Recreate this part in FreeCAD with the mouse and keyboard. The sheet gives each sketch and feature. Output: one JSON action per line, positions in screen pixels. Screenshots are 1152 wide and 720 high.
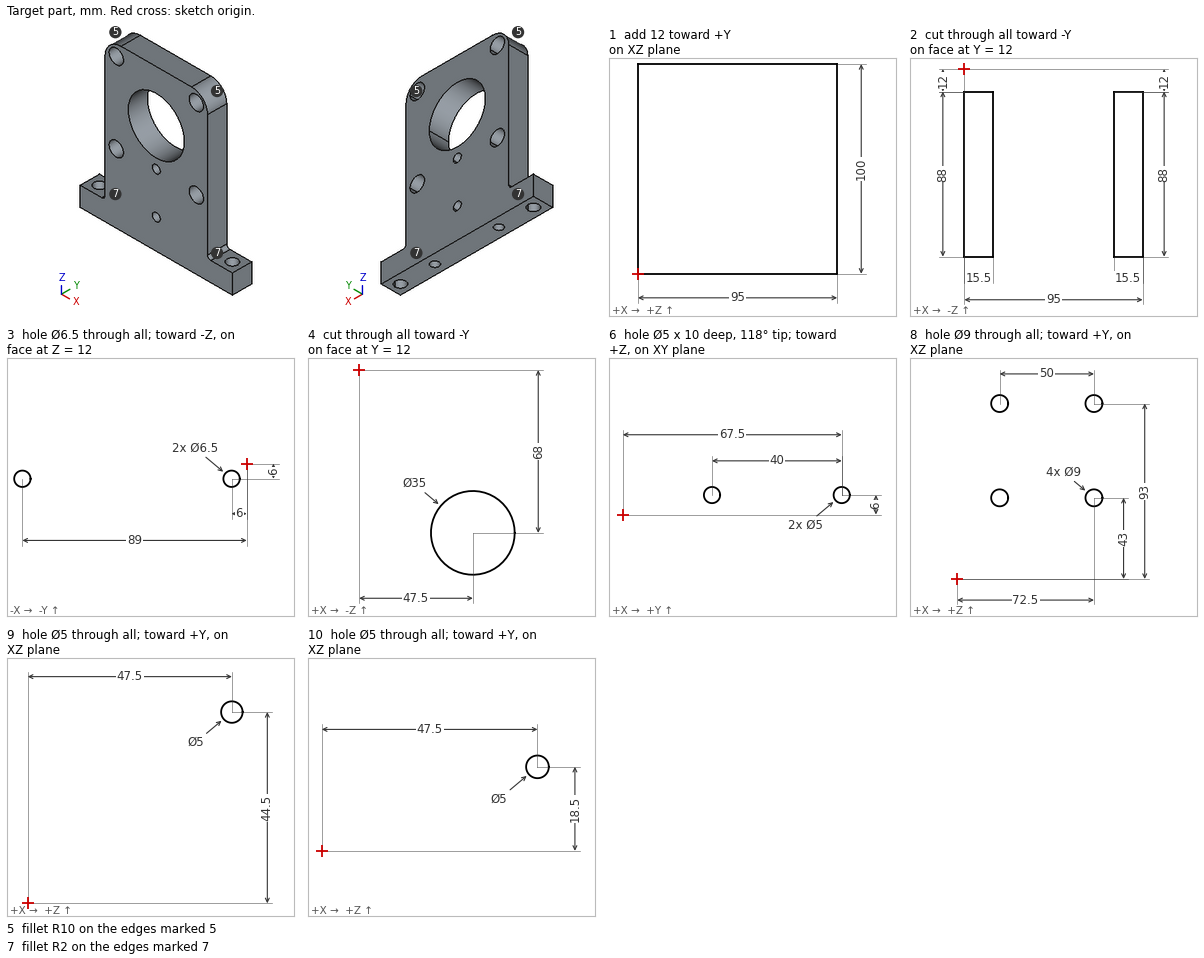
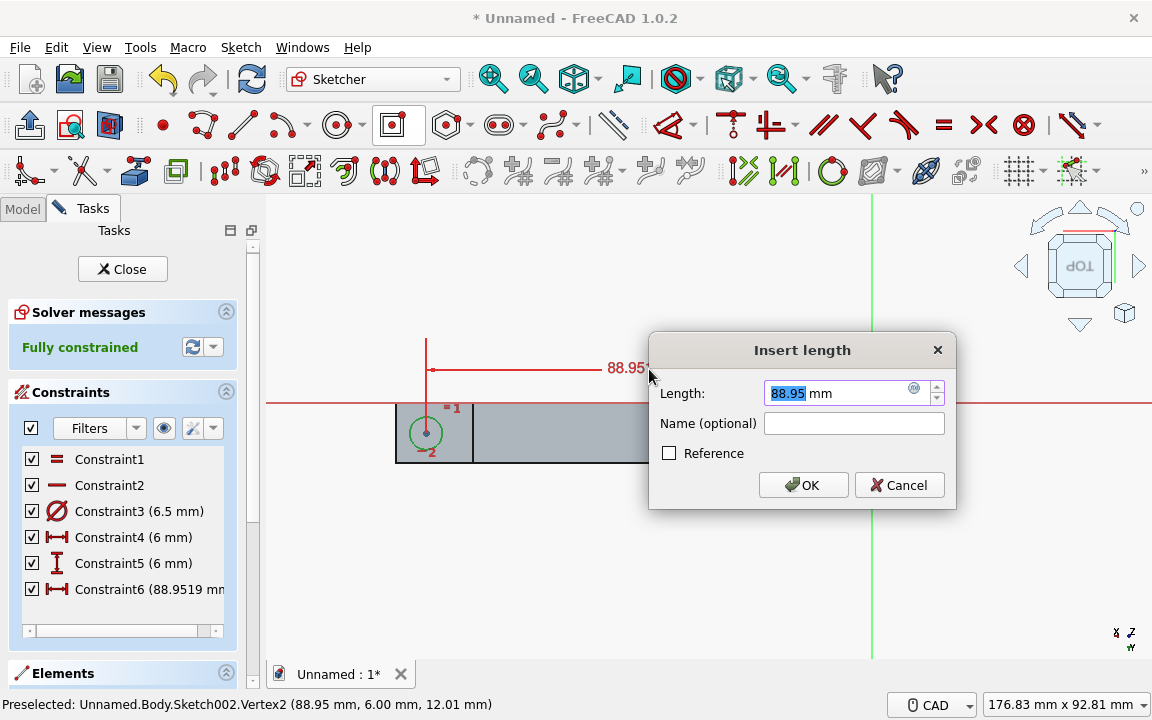
{"action": "type", "text": "89"}
{"action": "key", "text": "Return"}
{"action": "key", "text": "Escape"}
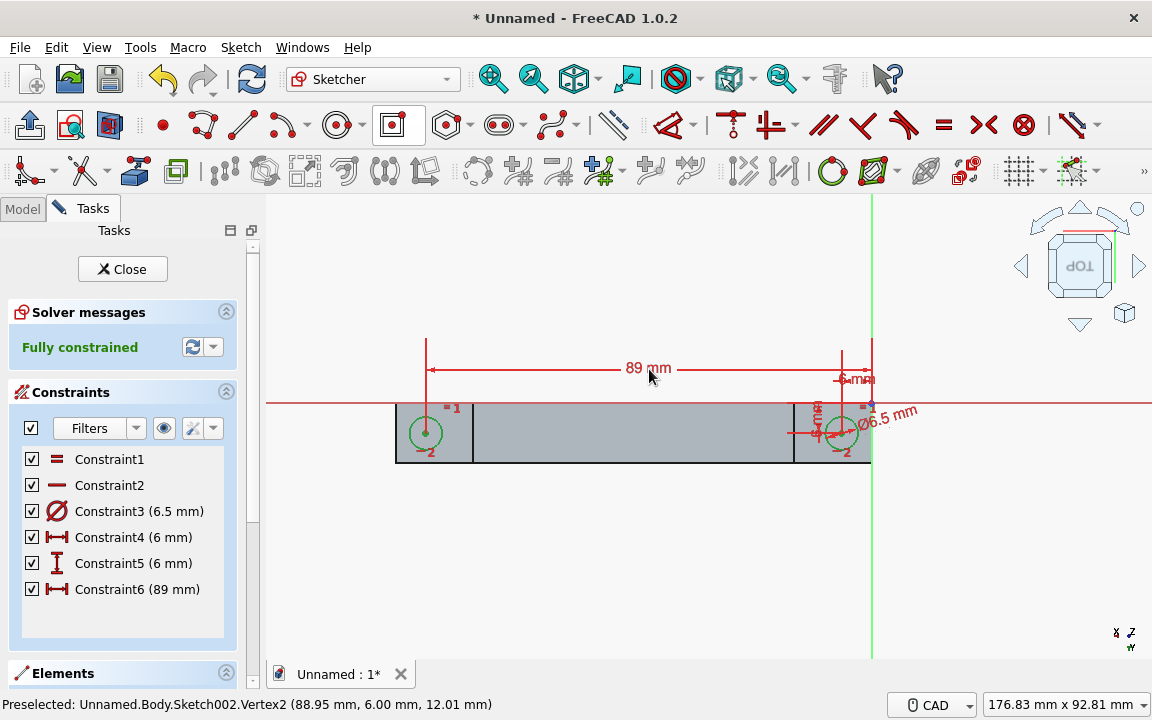
{"action": "left_click", "coordinate": [123, 269]}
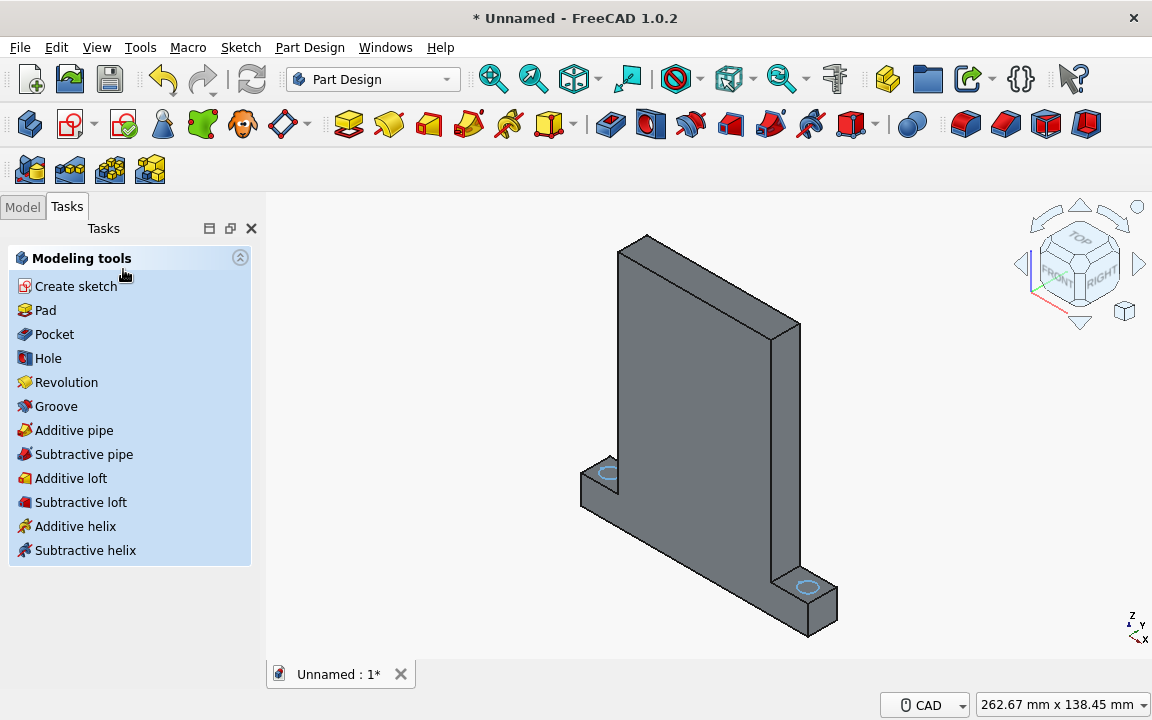
{"action": "left_click", "coordinate": [652, 124]}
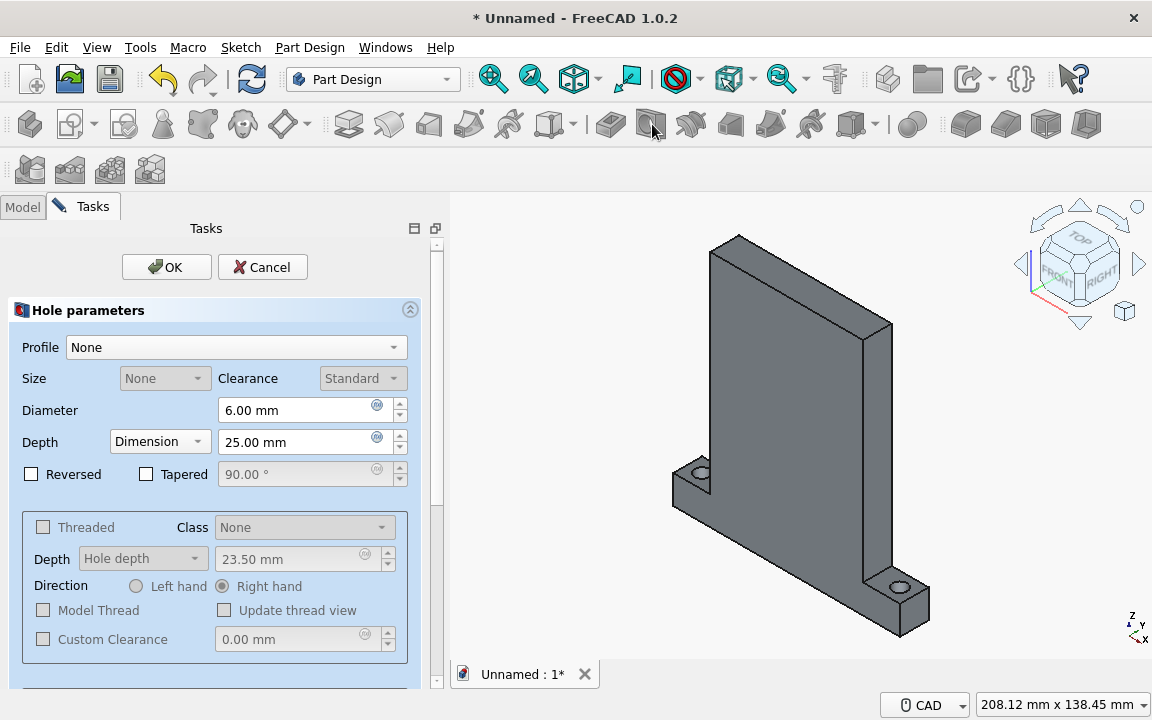
{"action": "triple_click", "coordinate": [305, 410]}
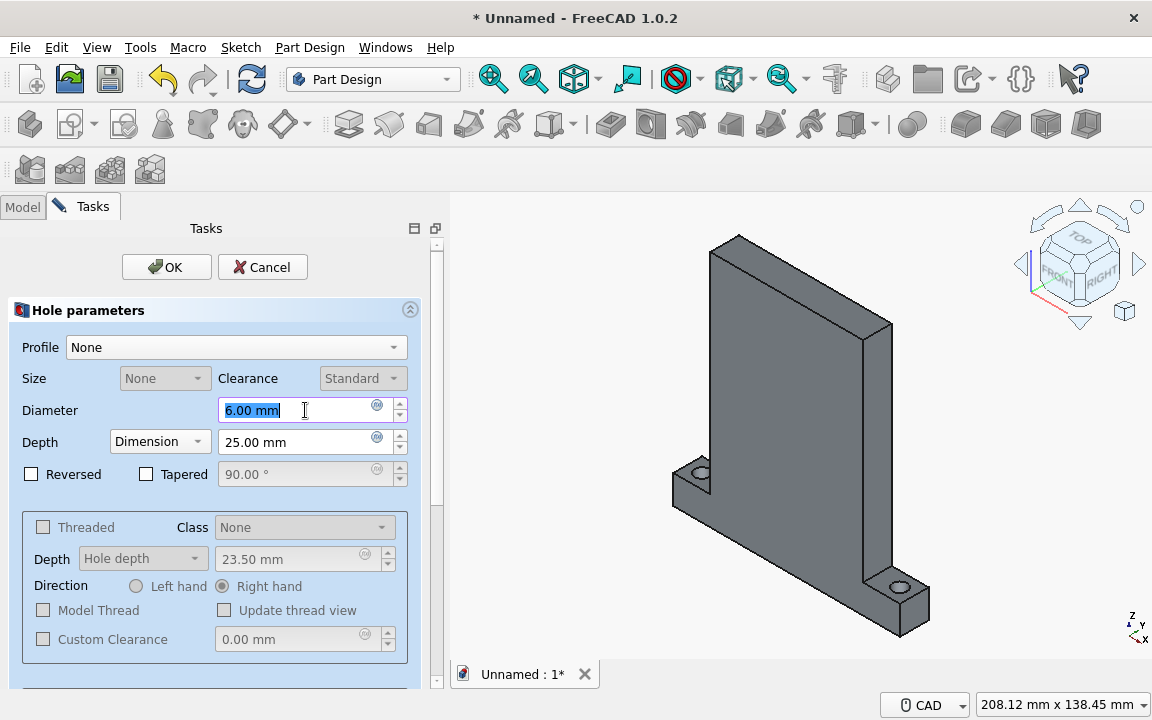
{"action": "type", "text": "6.5"}
{"action": "key", "text": "Tab"}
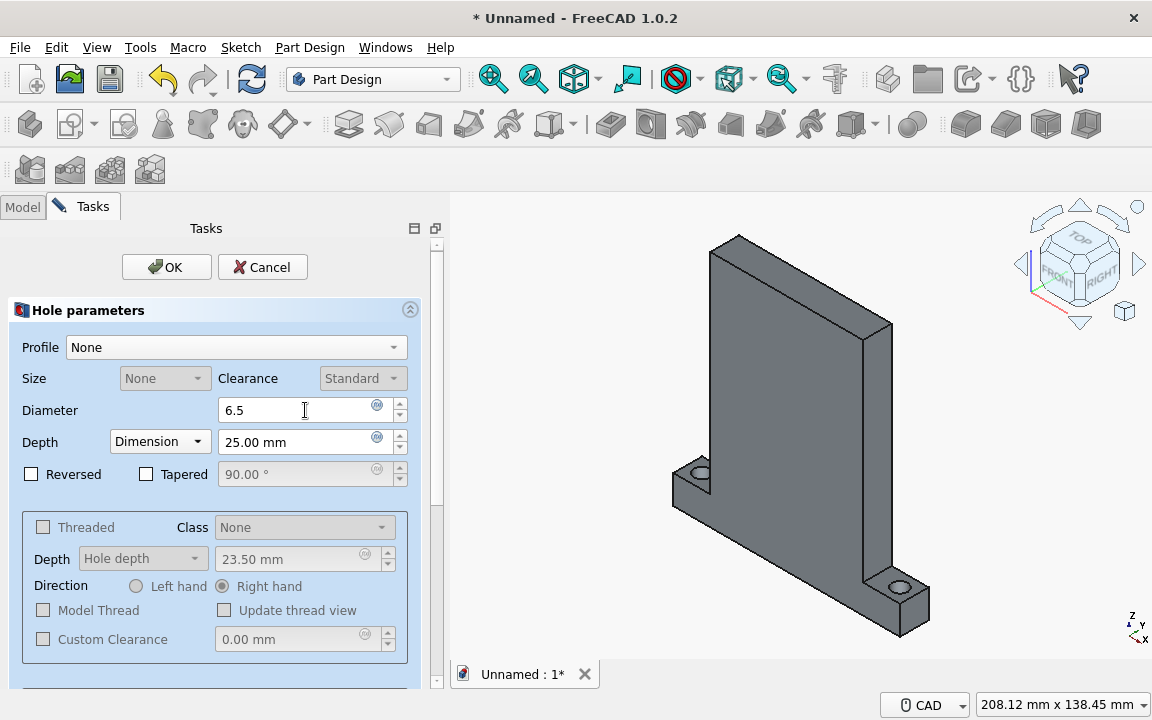
{"action": "left_click", "coordinate": [161, 442]}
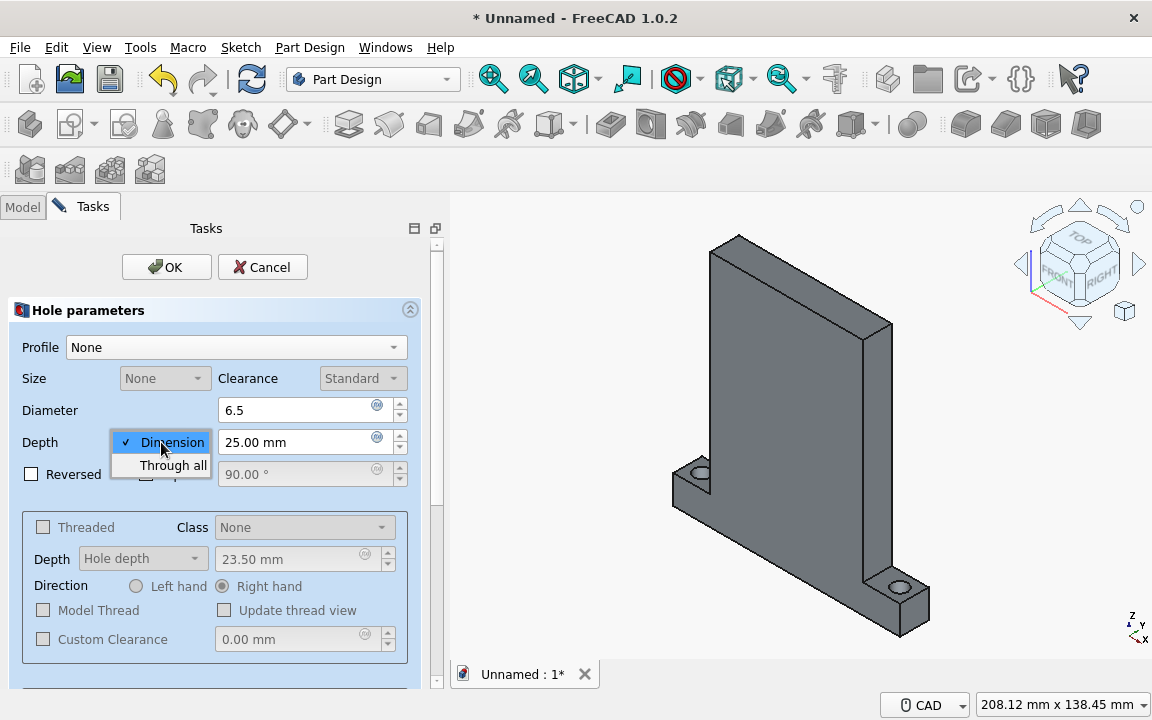
{"action": "left_click", "coordinate": [160, 466]}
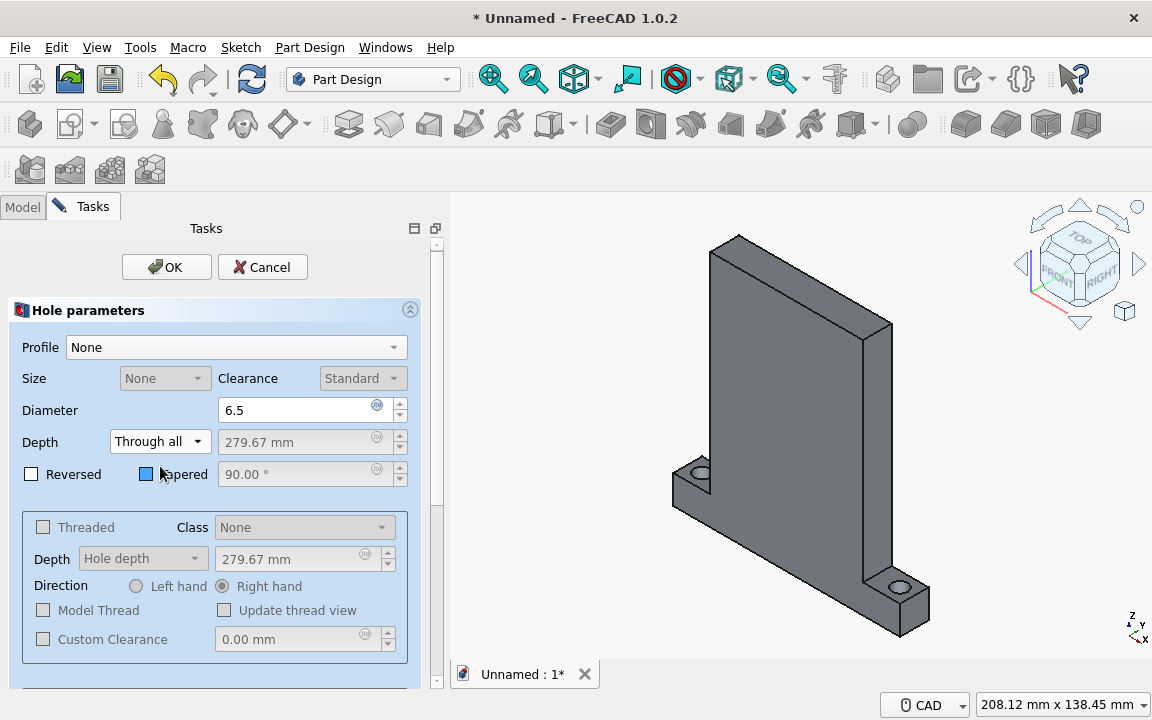
{"action": "left_click", "coordinate": [167, 267]}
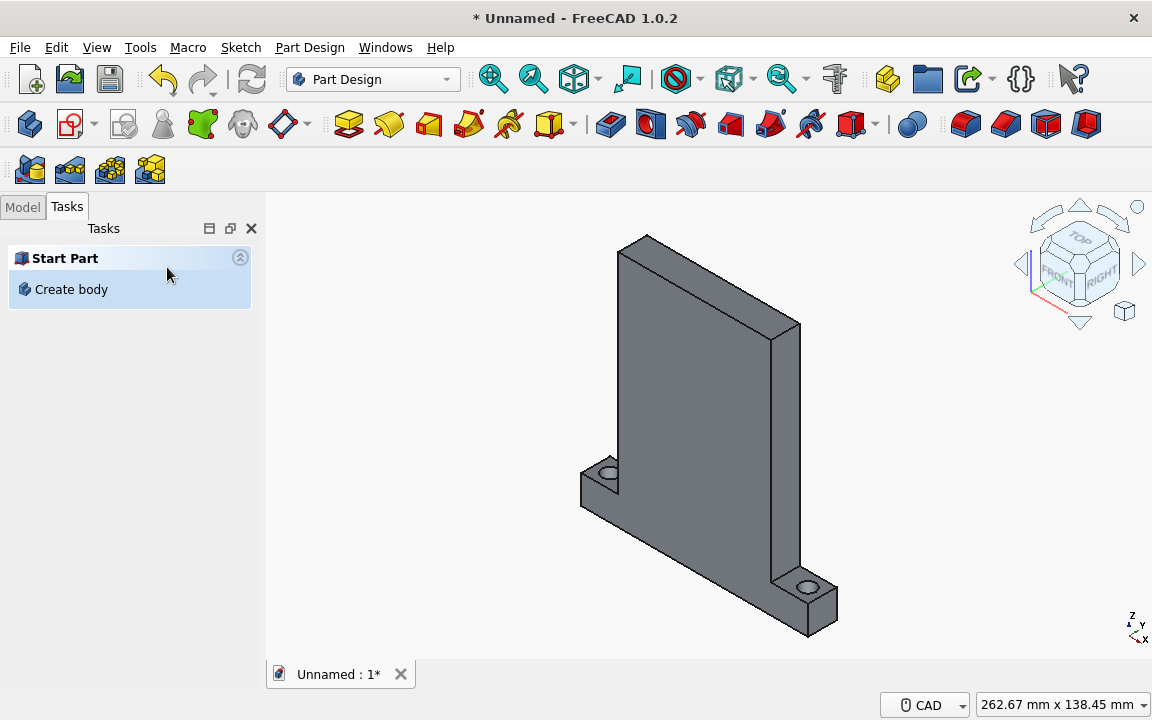
{"action": "key", "text": "4"}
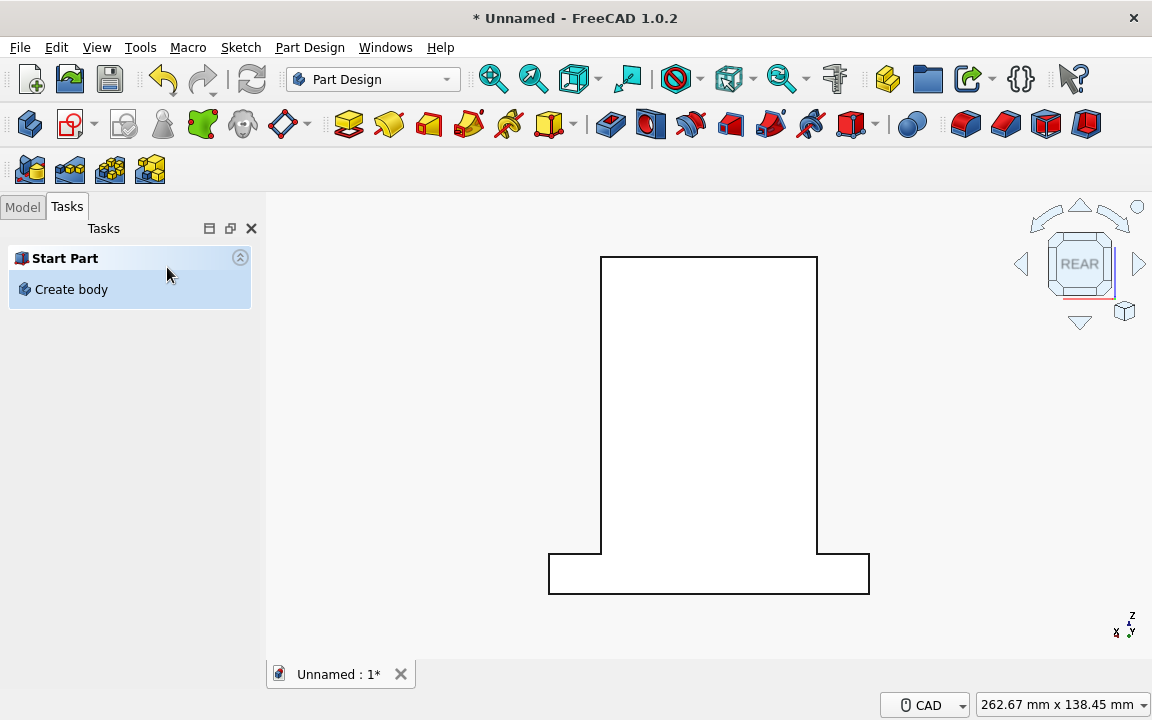
{"action": "left_click", "coordinate": [709, 376]}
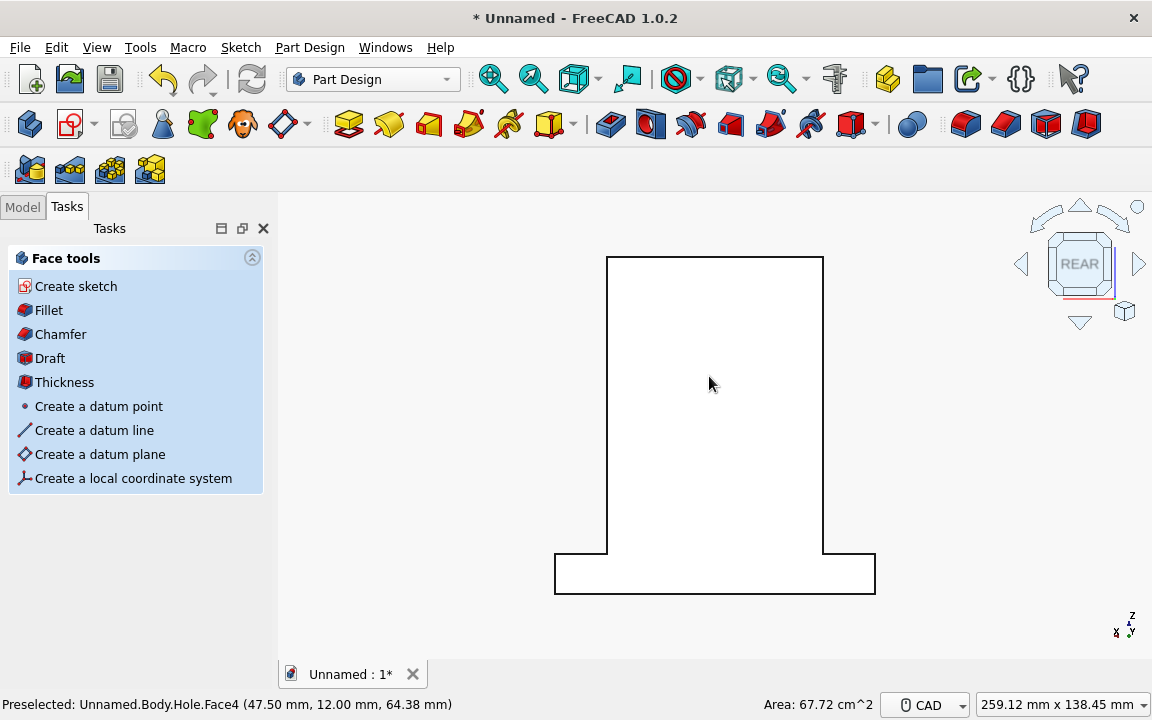
{"action": "left_click", "coordinate": [70, 124]}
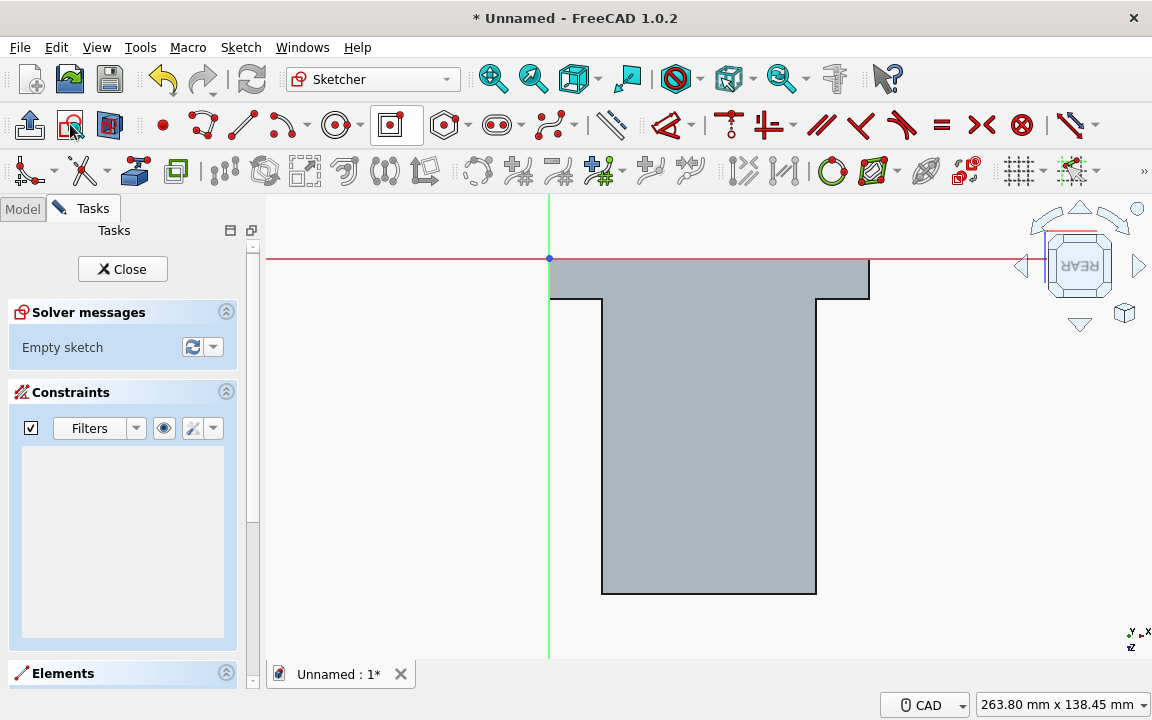
{"action": "left_click", "coordinate": [336, 126]}